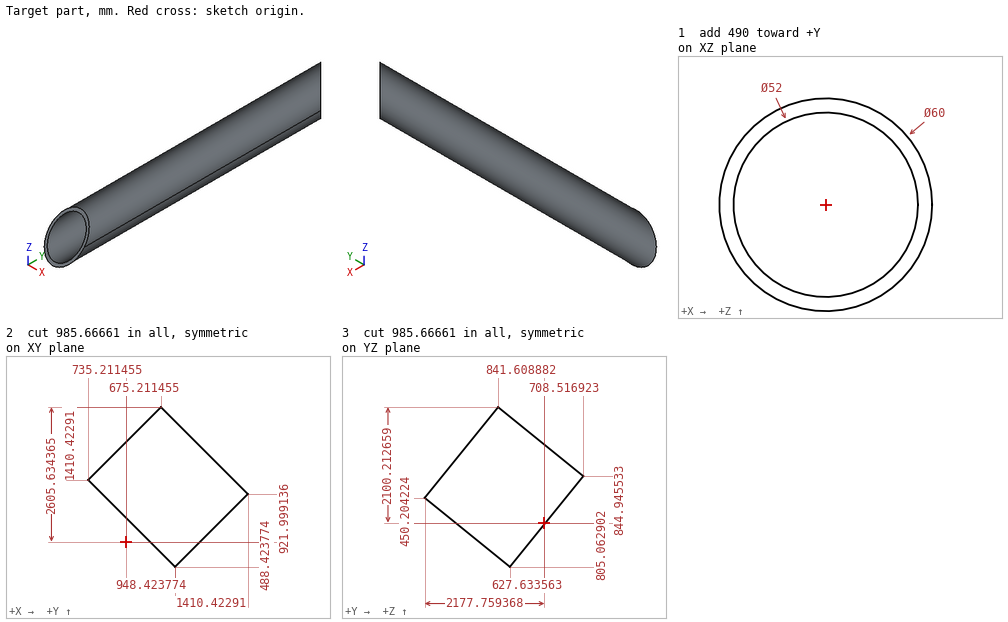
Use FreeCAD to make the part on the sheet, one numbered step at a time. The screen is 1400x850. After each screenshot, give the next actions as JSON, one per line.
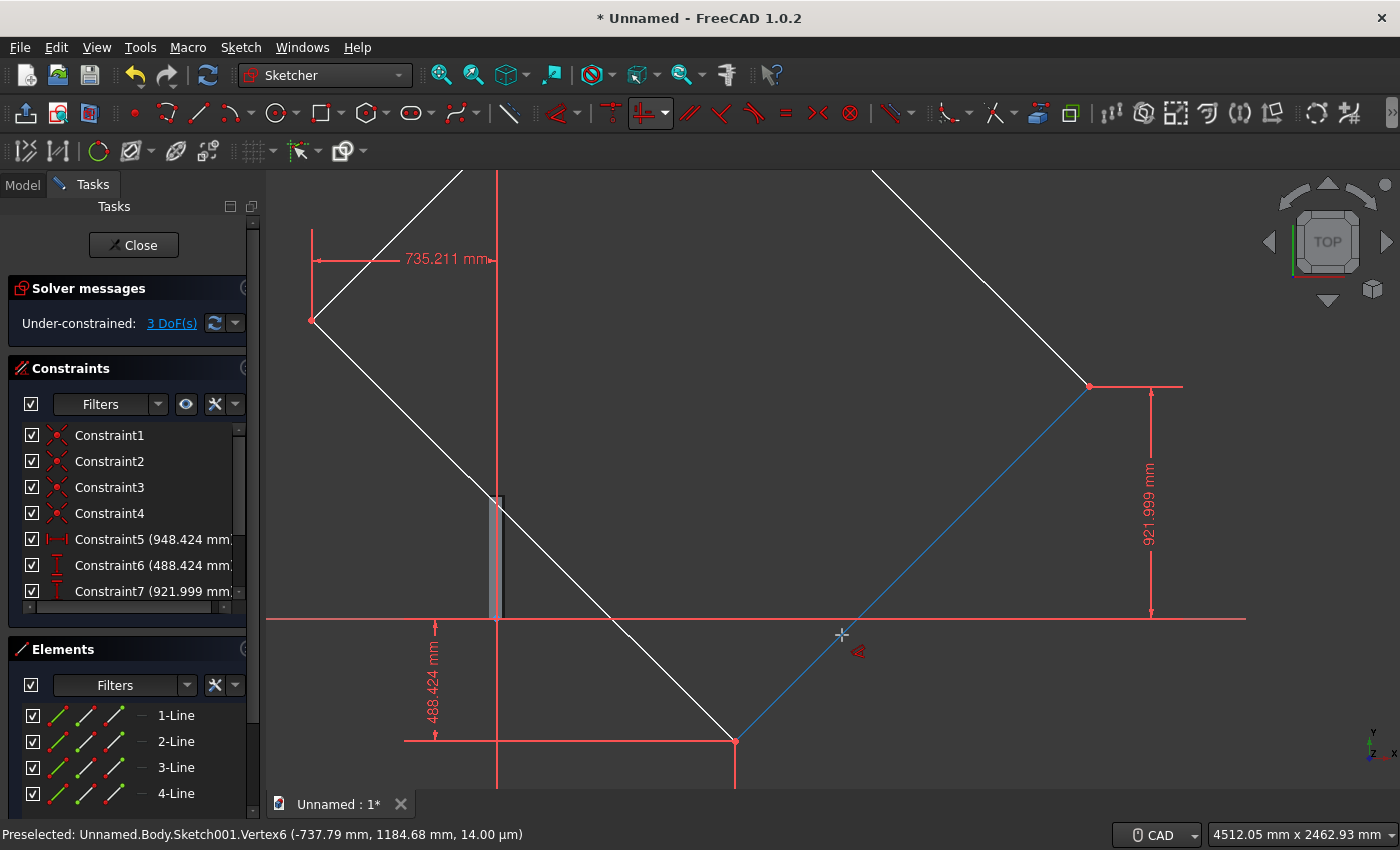
{"action": "left_click", "coordinate": [841, 635]}
{"action": "left_click", "coordinate": [912, 353]}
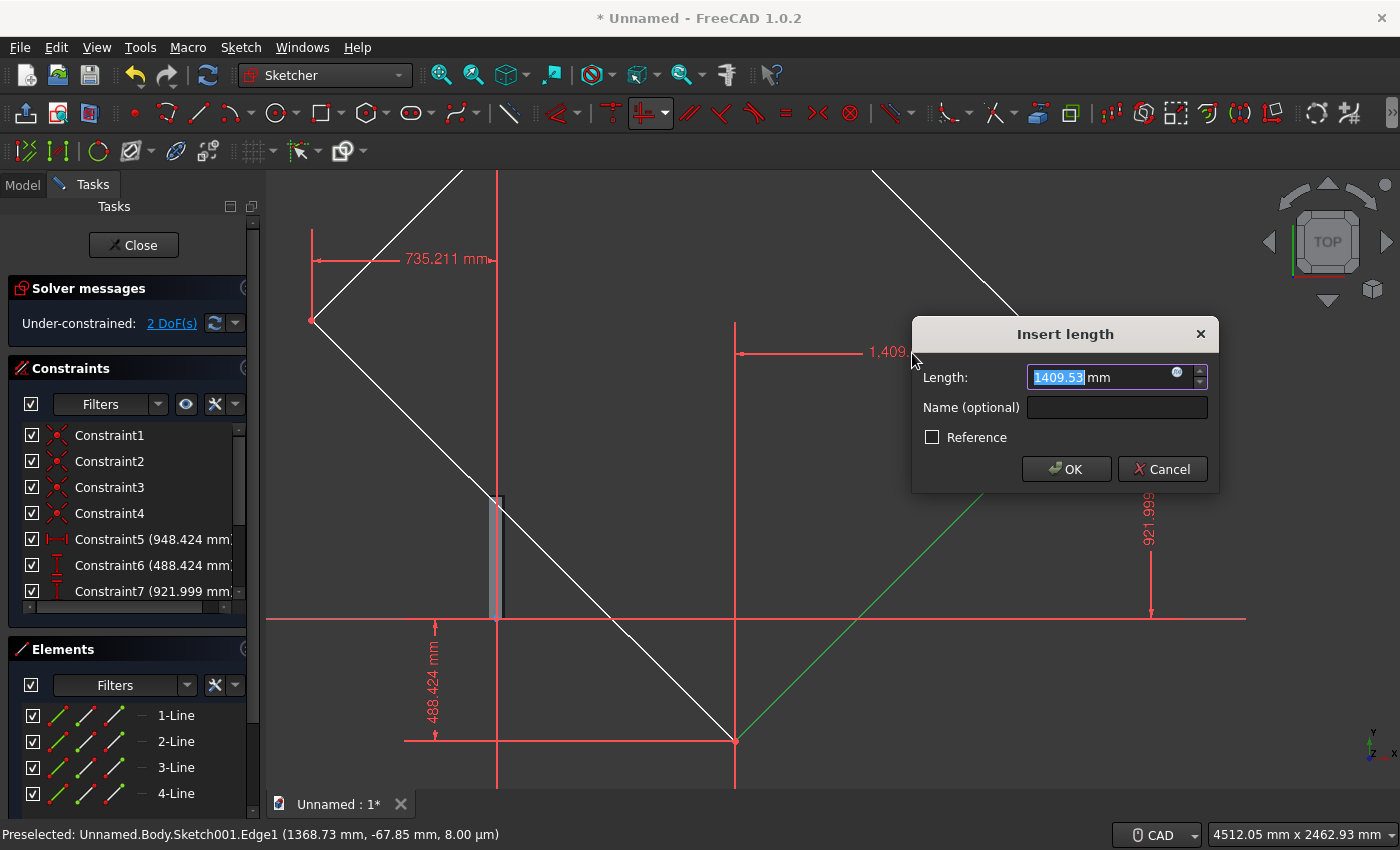
{"action": "type", "text": "1410.42291"}
{"action": "key", "text": "Return"}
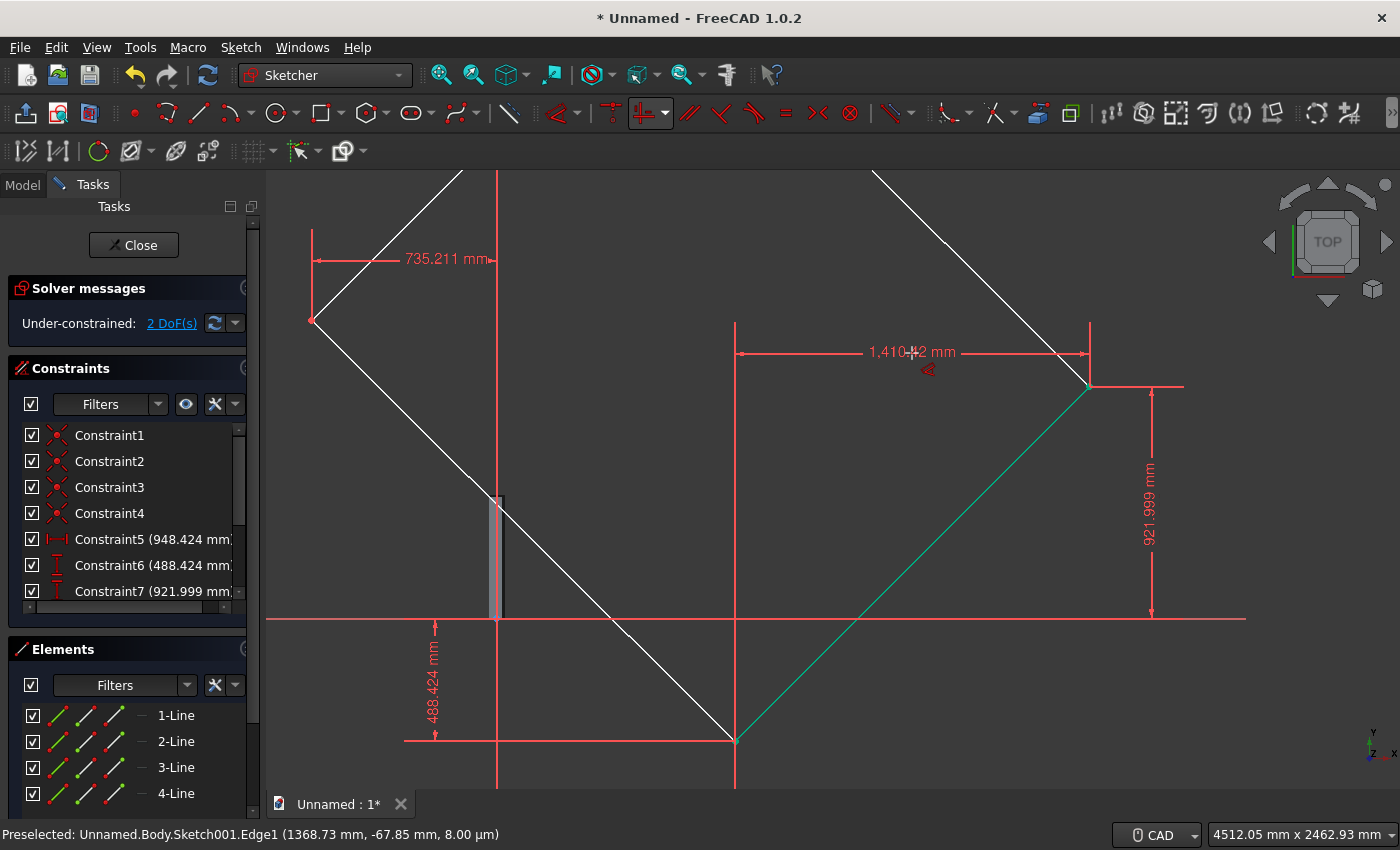
{"action": "left_click", "coordinate": [418, 214]}
{"action": "left_click", "coordinate": [700, 259]}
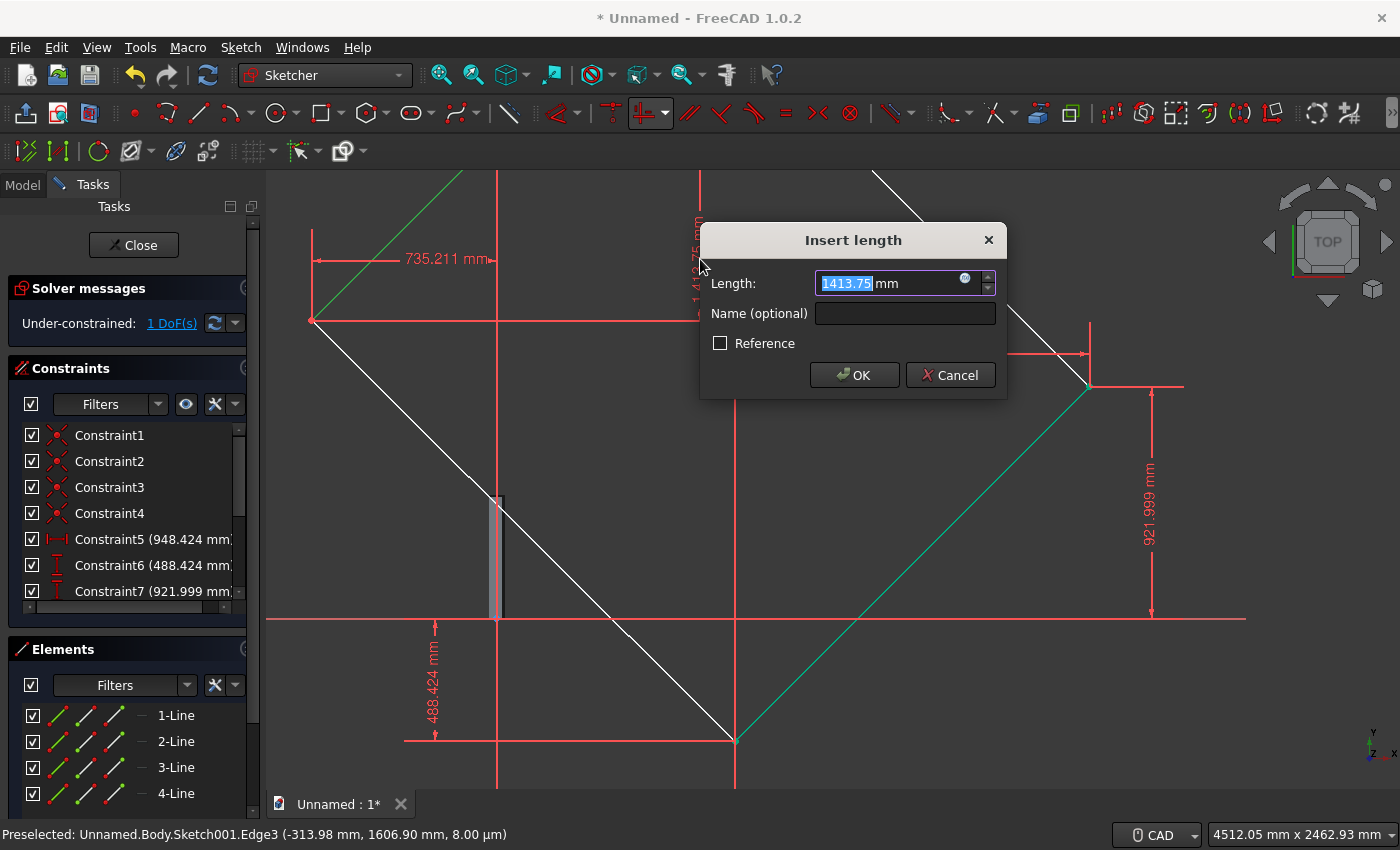
{"action": "type", "text": "1410.42291"}
{"action": "key", "text": "Return"}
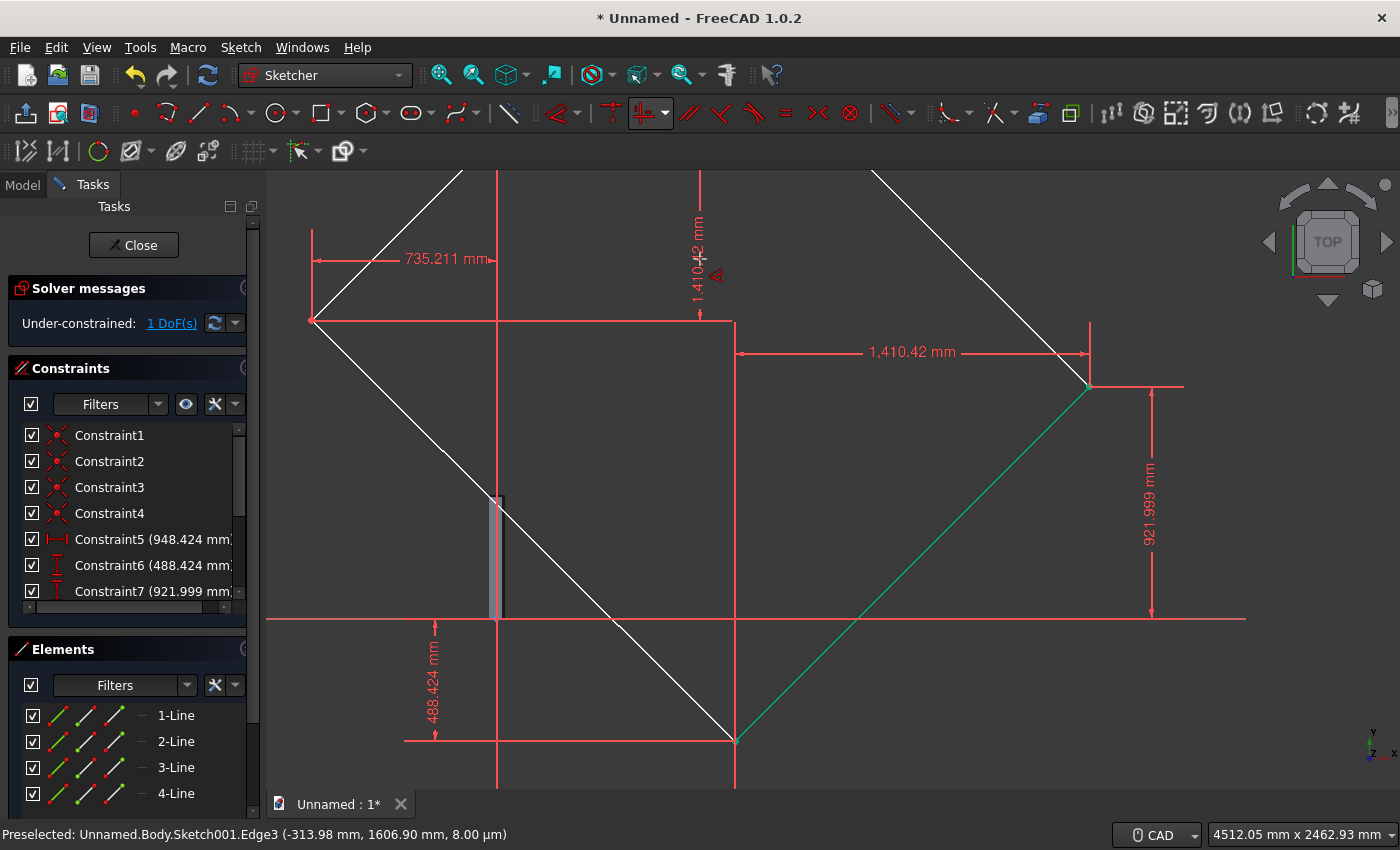
{"action": "scroll", "coordinate": [842, 634], "scroll_direction": "down", "scroll_amount": 3}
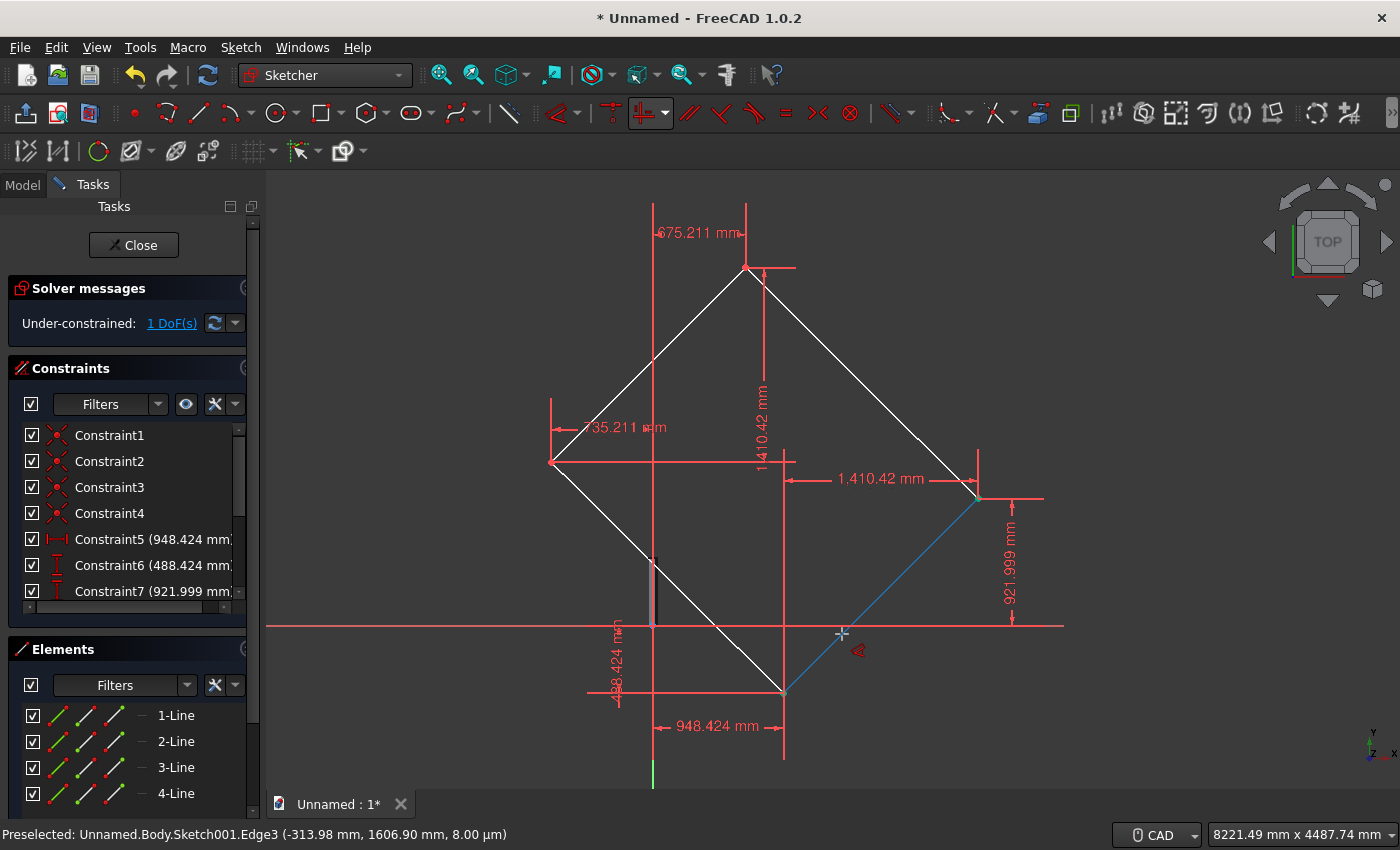
{"action": "left_click", "coordinate": [746, 268]}
{"action": "left_click", "coordinate": [619, 365]}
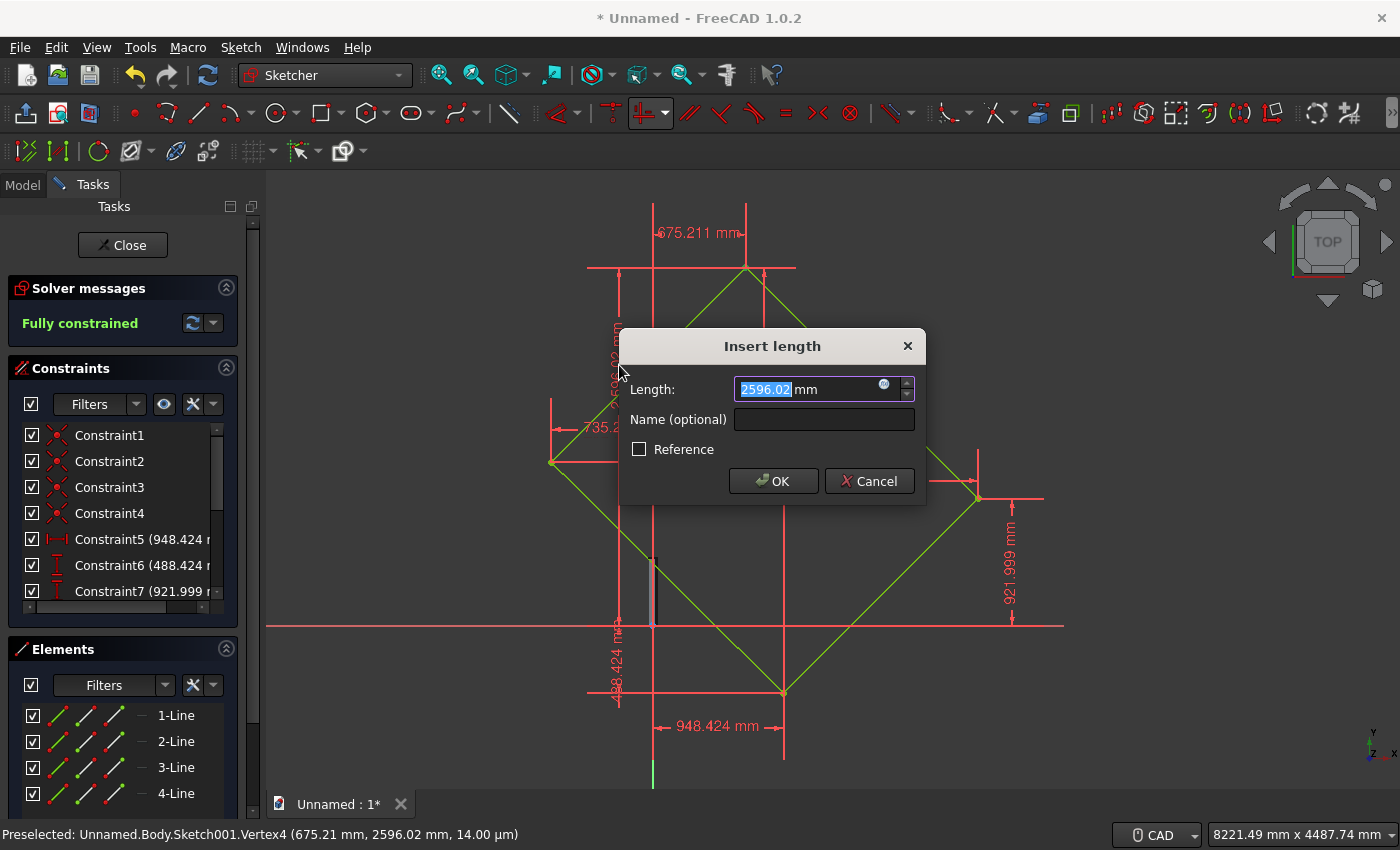
{"action": "type", "text": "2605.634365"}
{"action": "key", "text": "Return"}
{"action": "key", "text": "Escape"}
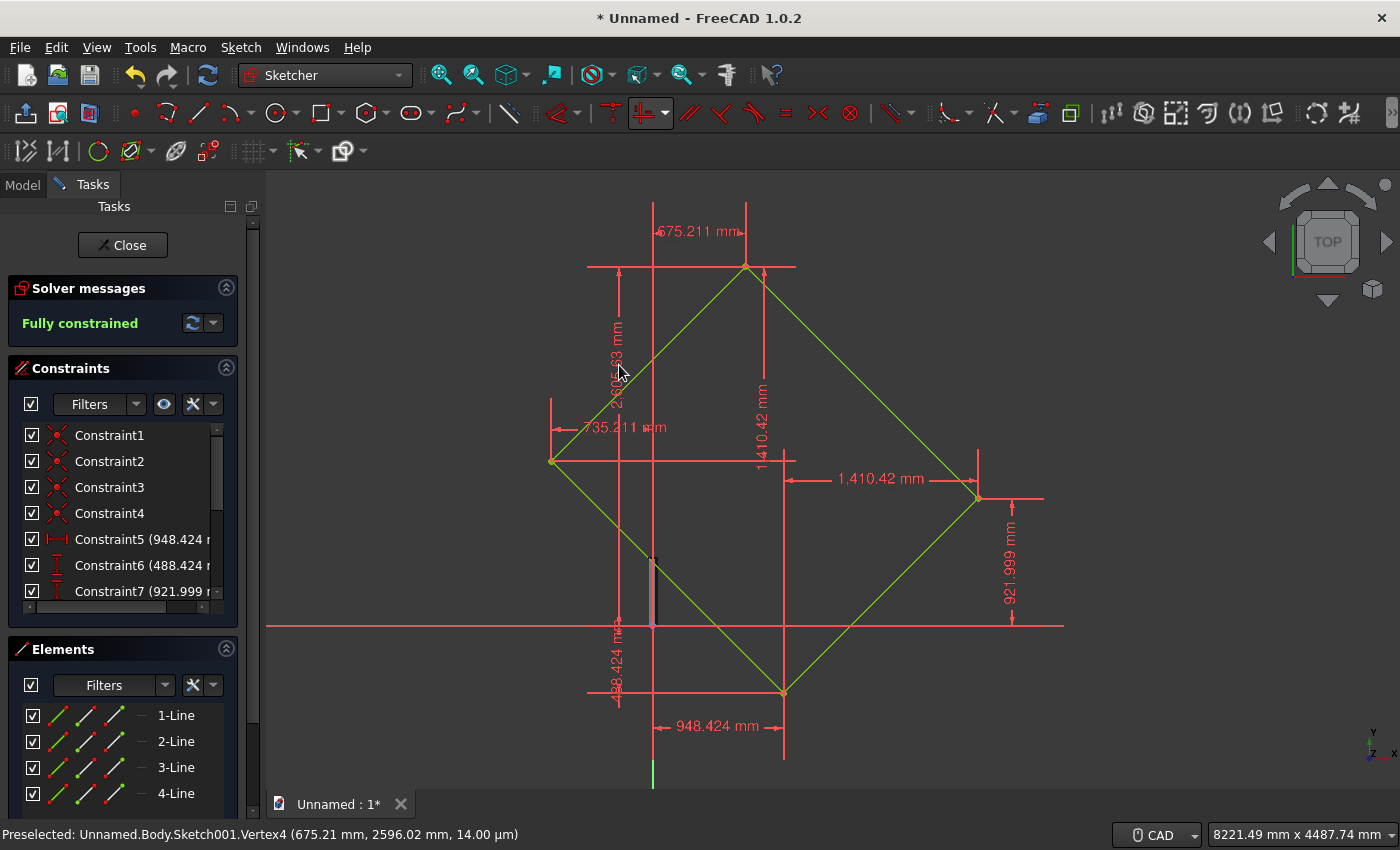
{"action": "left_click", "coordinate": [123, 245]}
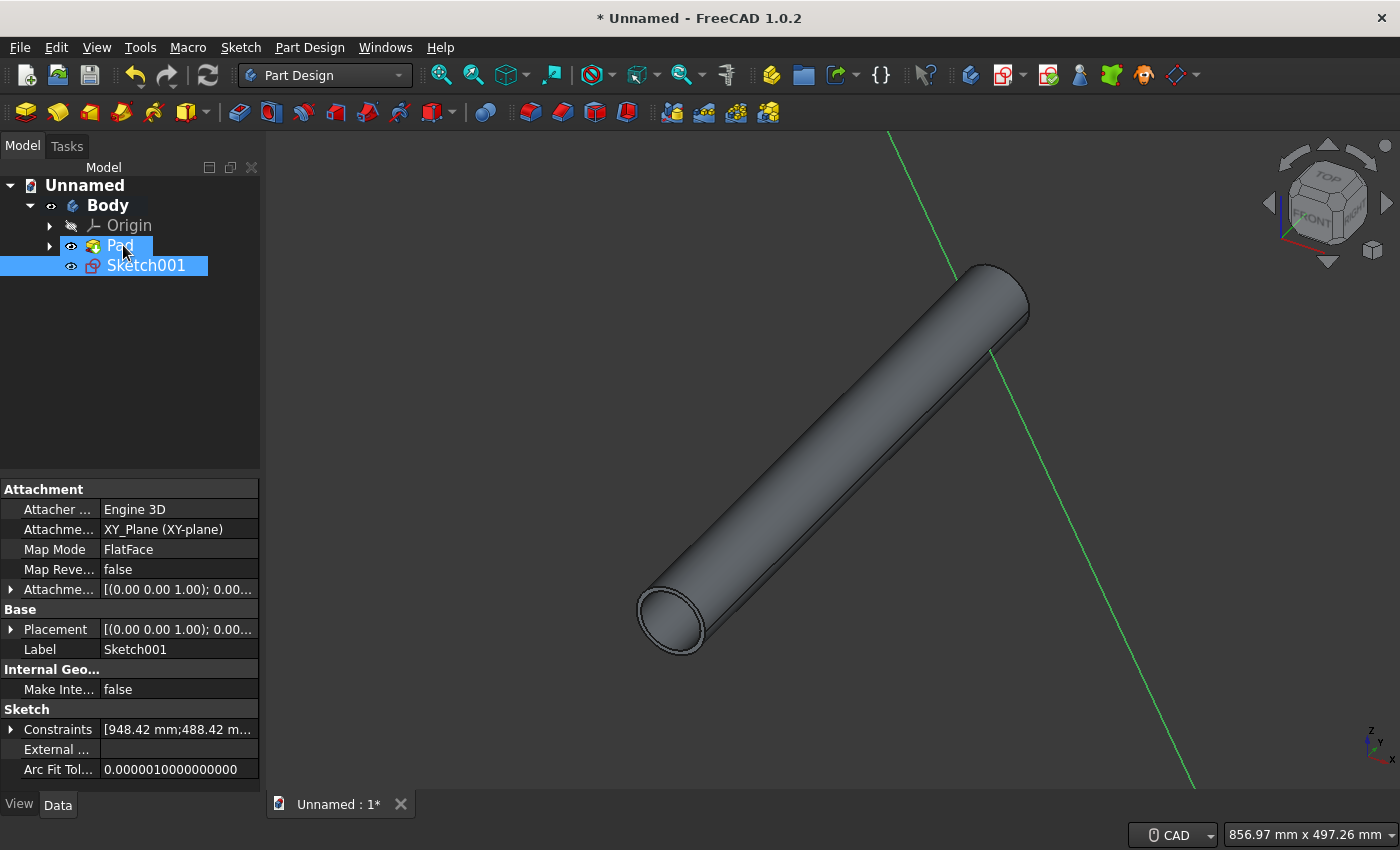
{"action": "left_click", "coordinate": [240, 112]}